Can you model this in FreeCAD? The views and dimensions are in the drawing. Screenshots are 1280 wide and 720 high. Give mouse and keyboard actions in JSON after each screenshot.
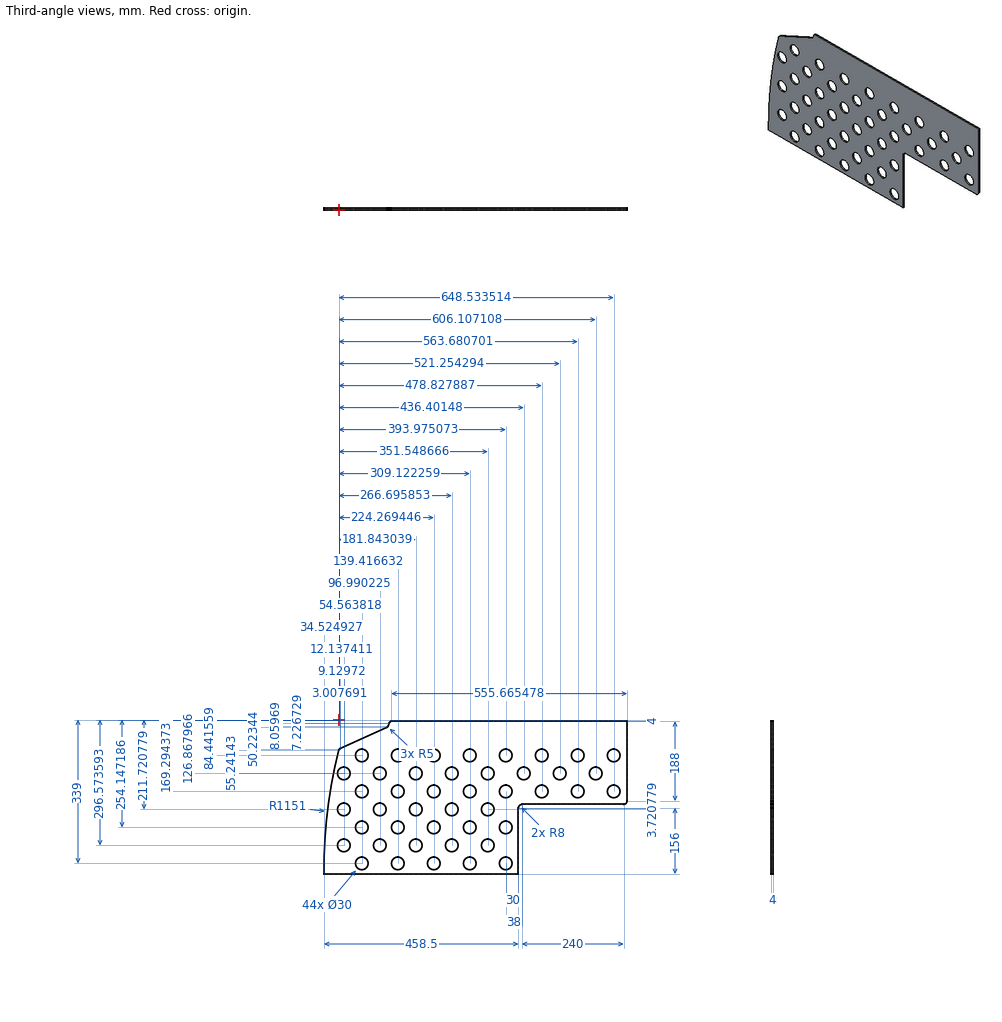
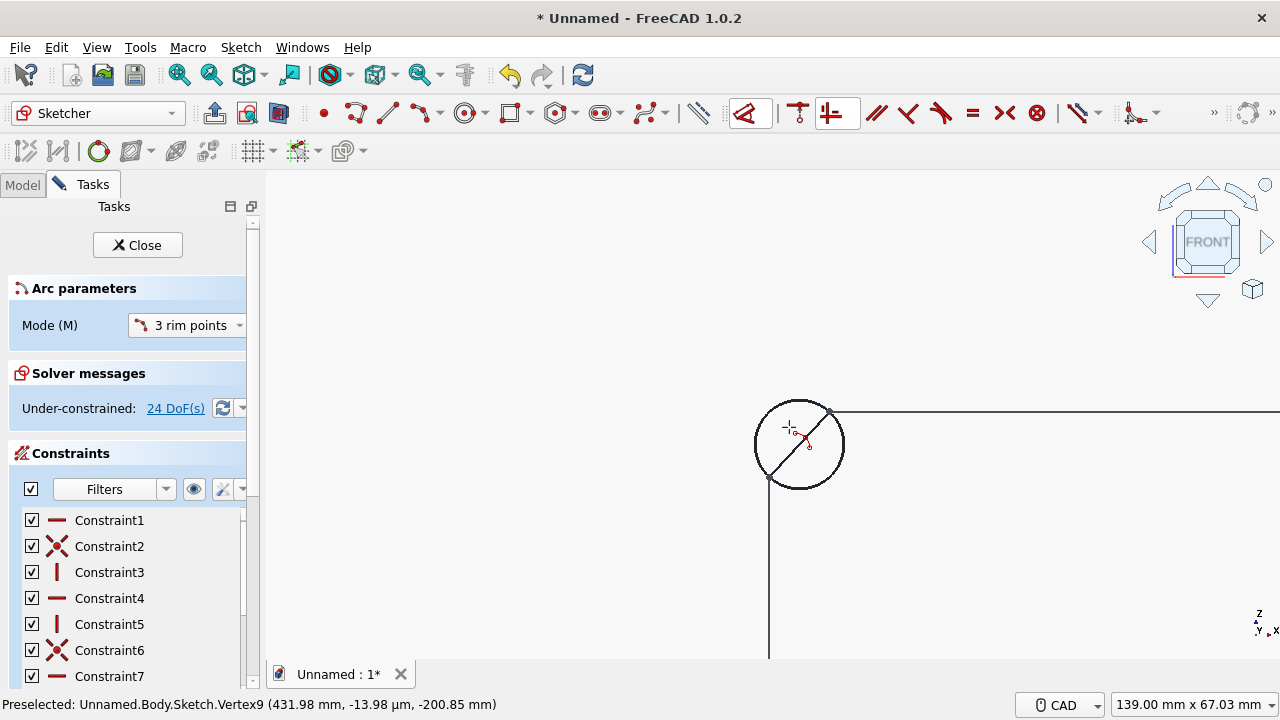
{"action": "left_click", "coordinate": [788, 423]}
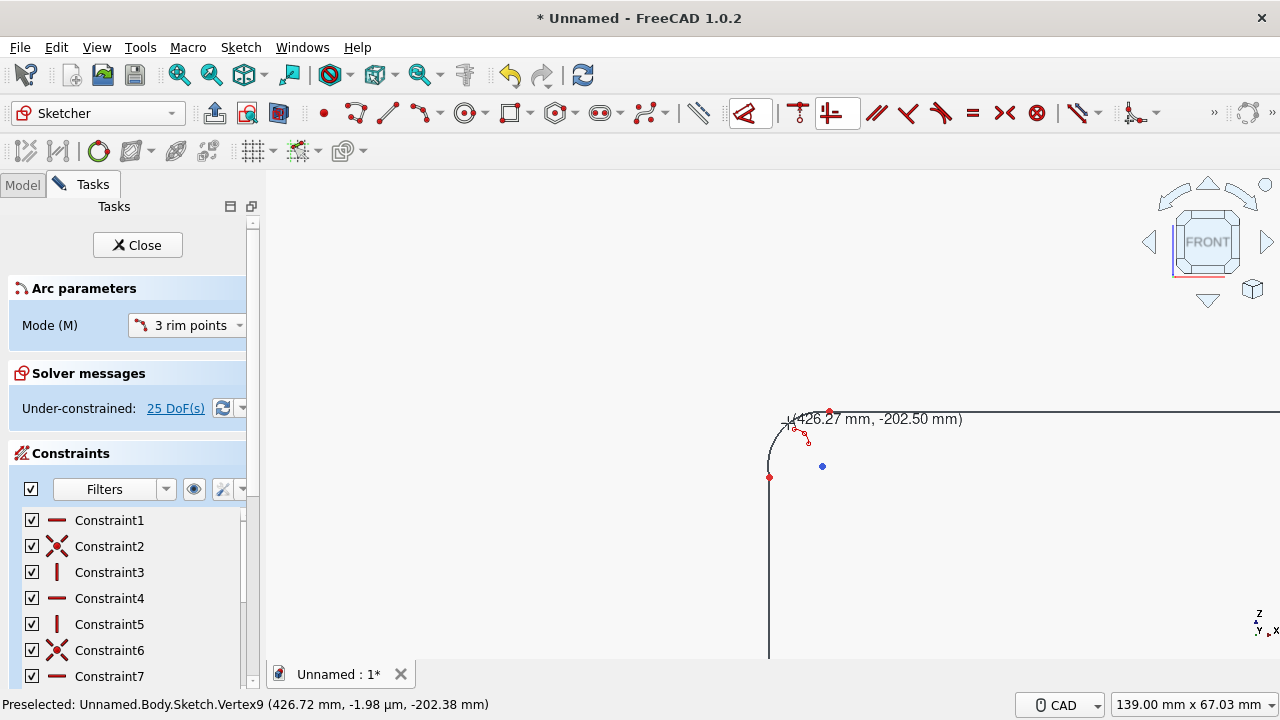
{"action": "scroll", "coordinate": [788, 432], "scroll_direction": "down", "scroll_amount": 11}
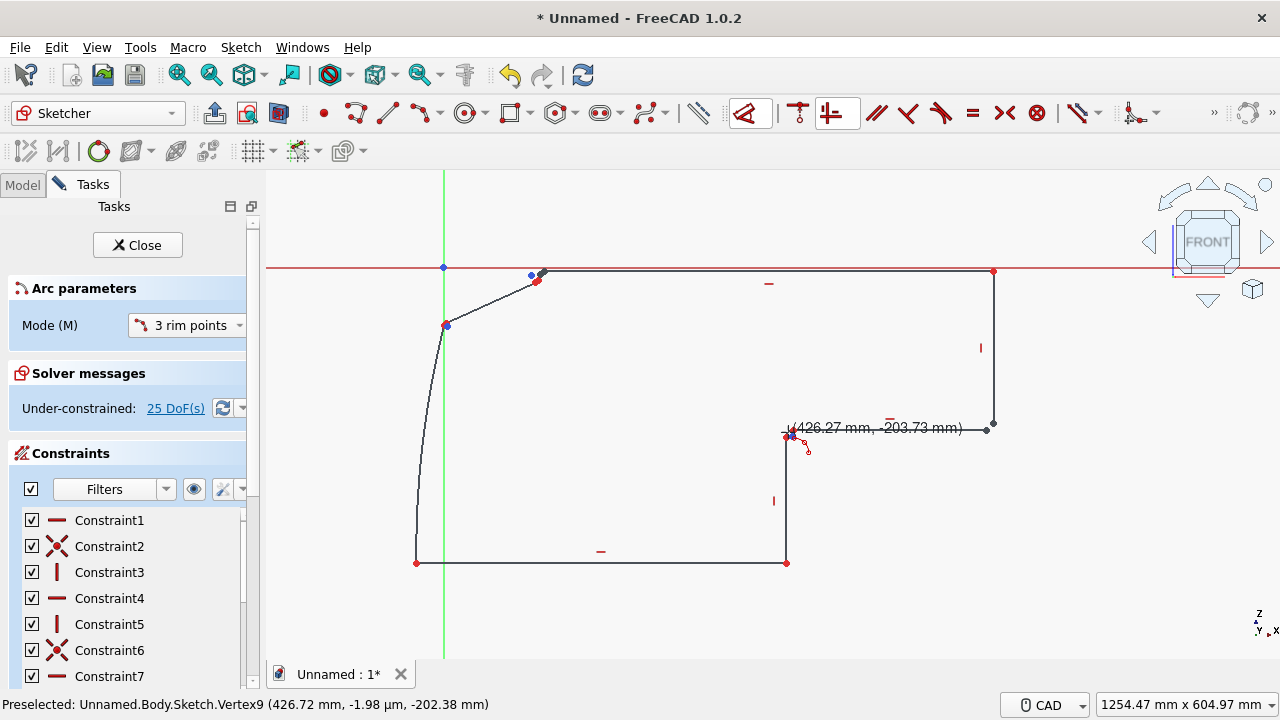
{"action": "scroll", "coordinate": [987, 430], "scroll_direction": "up", "scroll_amount": 3}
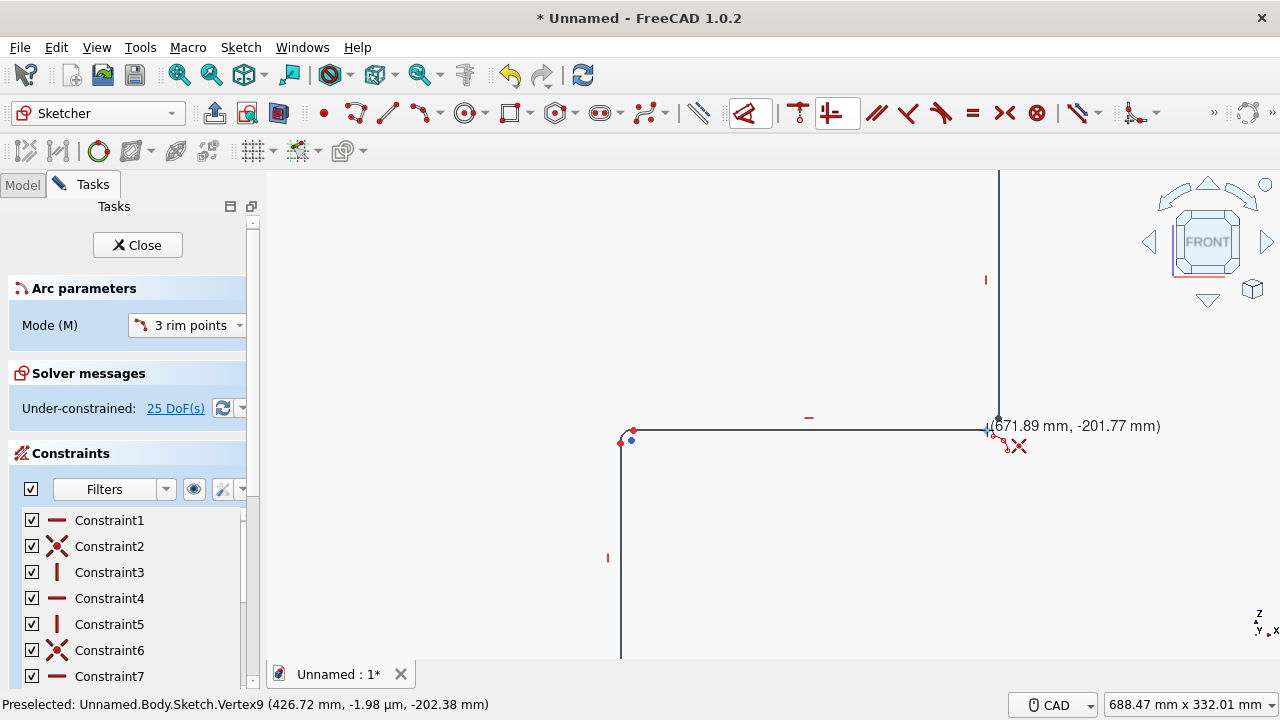
{"action": "left_click", "coordinate": [986, 430]}
{"action": "left_click", "coordinate": [999, 418]}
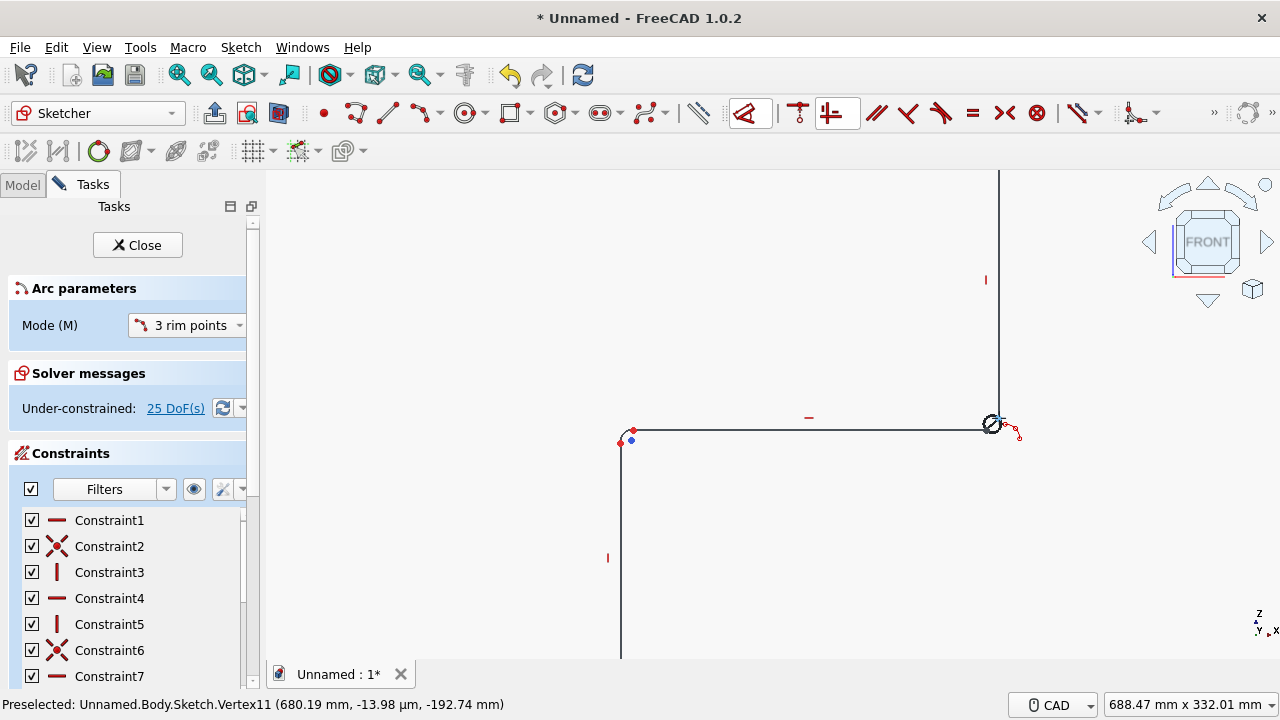
{"action": "scroll", "coordinate": [995, 425], "scroll_direction": "up", "scroll_amount": 8}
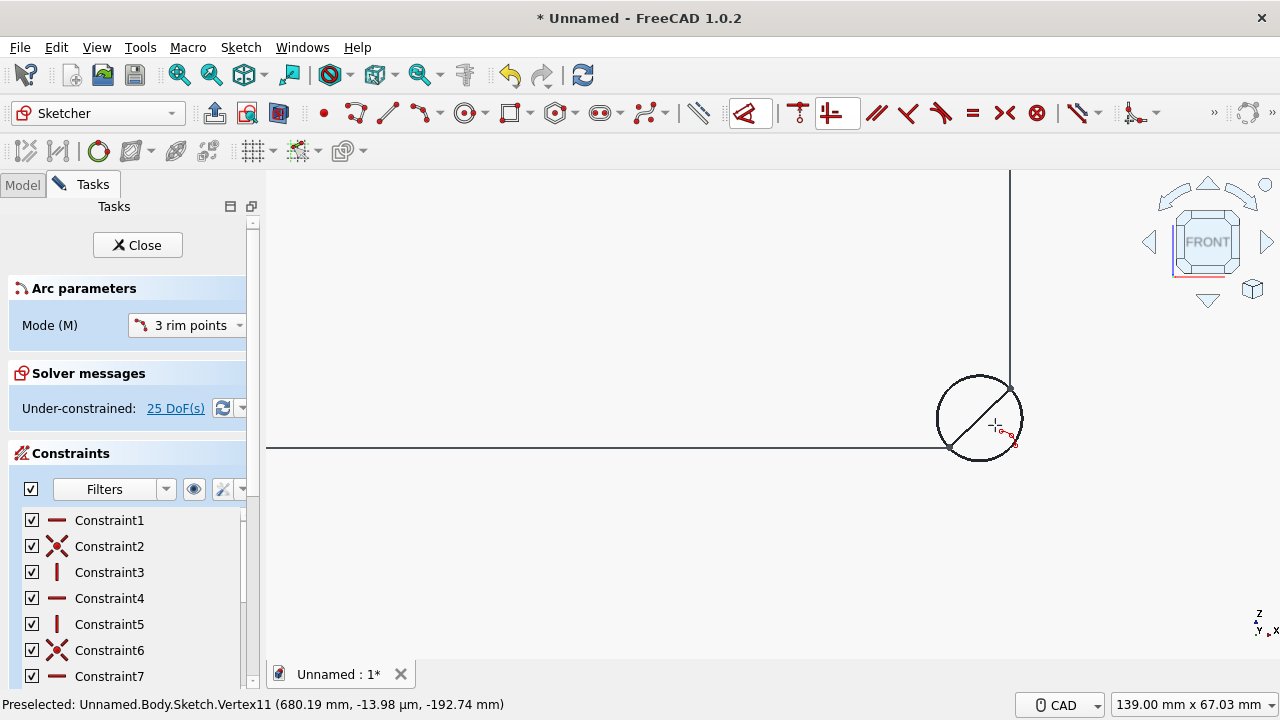
{"action": "left_click", "coordinate": [992, 425]}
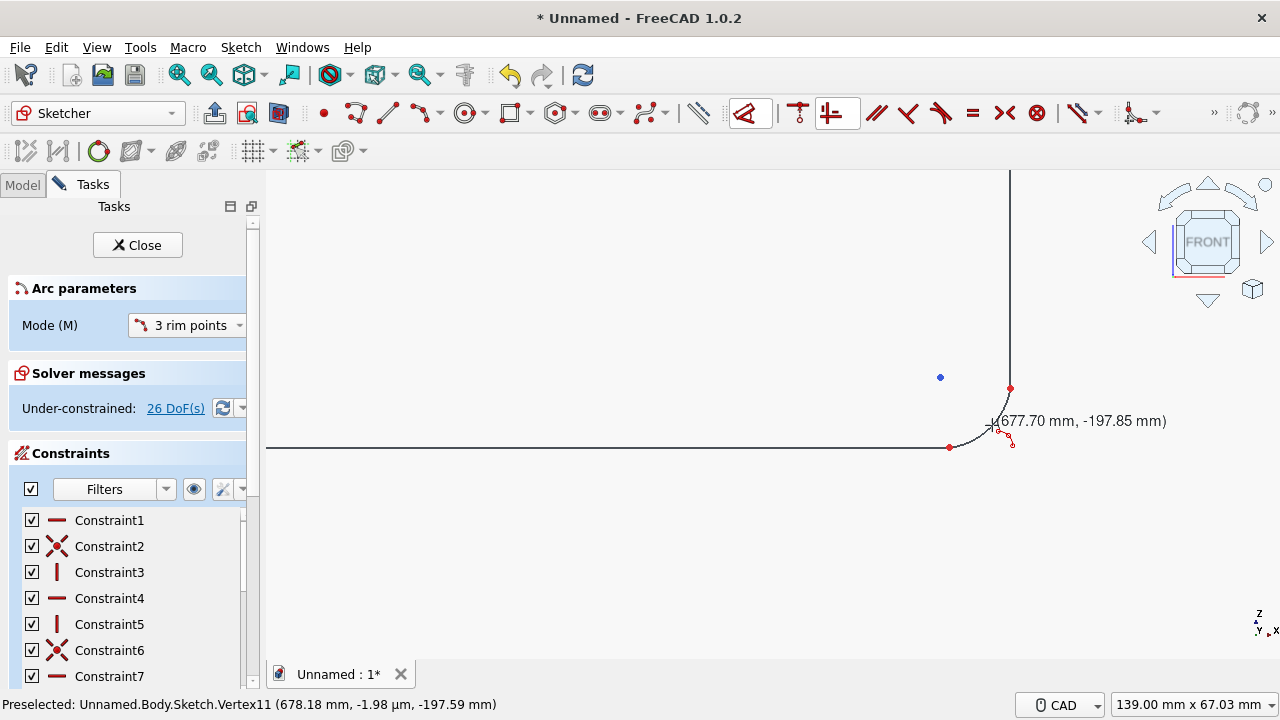
{"action": "scroll", "coordinate": [991, 427], "scroll_direction": "down", "scroll_amount": 11}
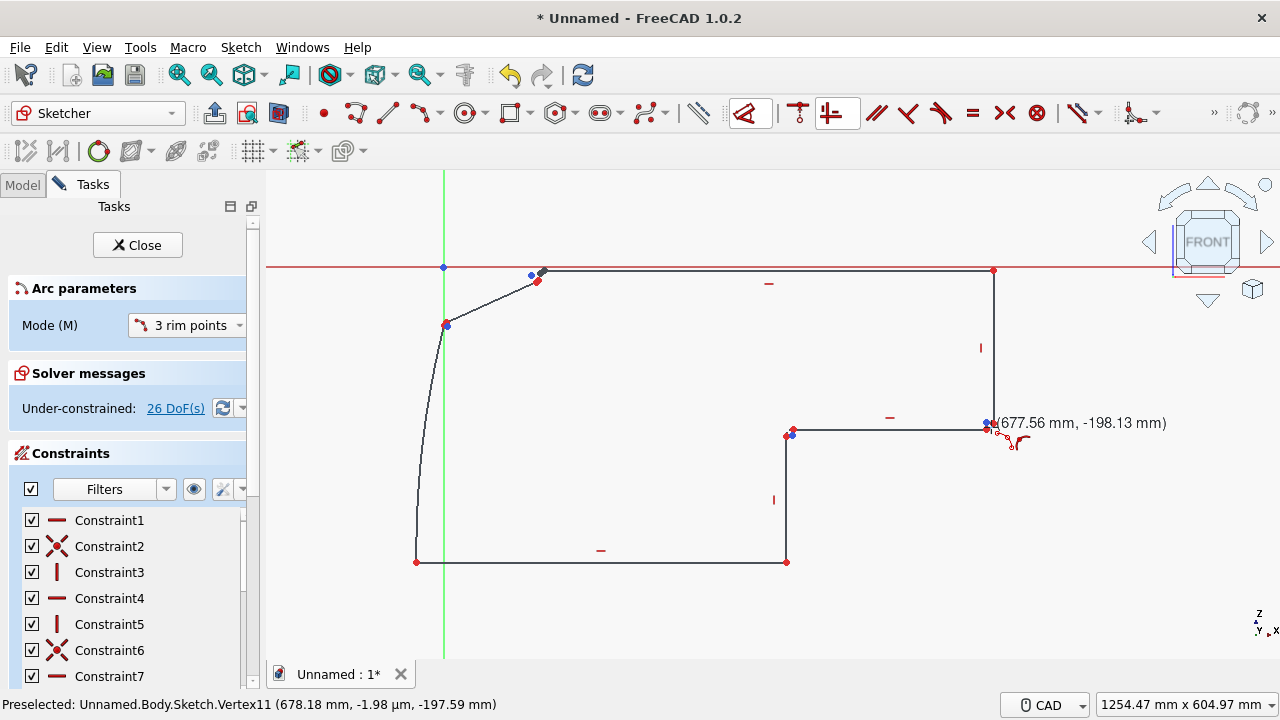
{"action": "scroll", "coordinate": [544, 271], "scroll_direction": "up", "scroll_amount": 8}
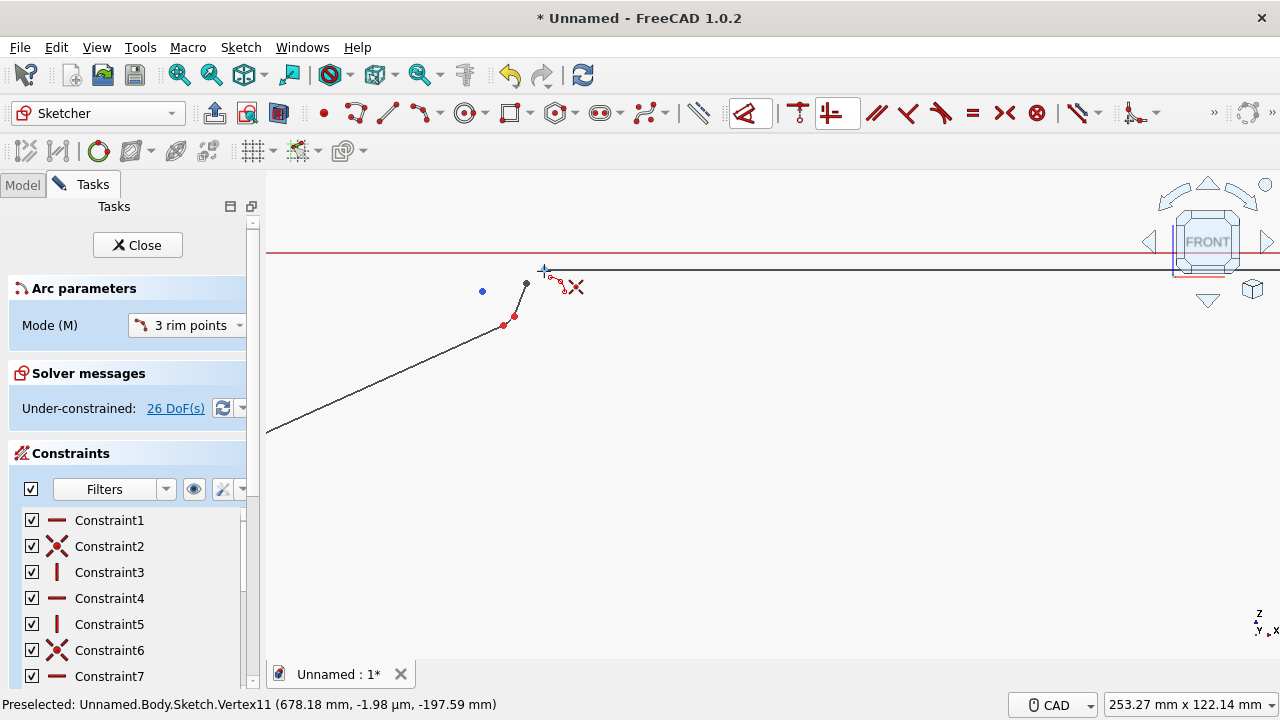
{"action": "left_click", "coordinate": [545, 270]}
{"action": "left_click", "coordinate": [527, 283]}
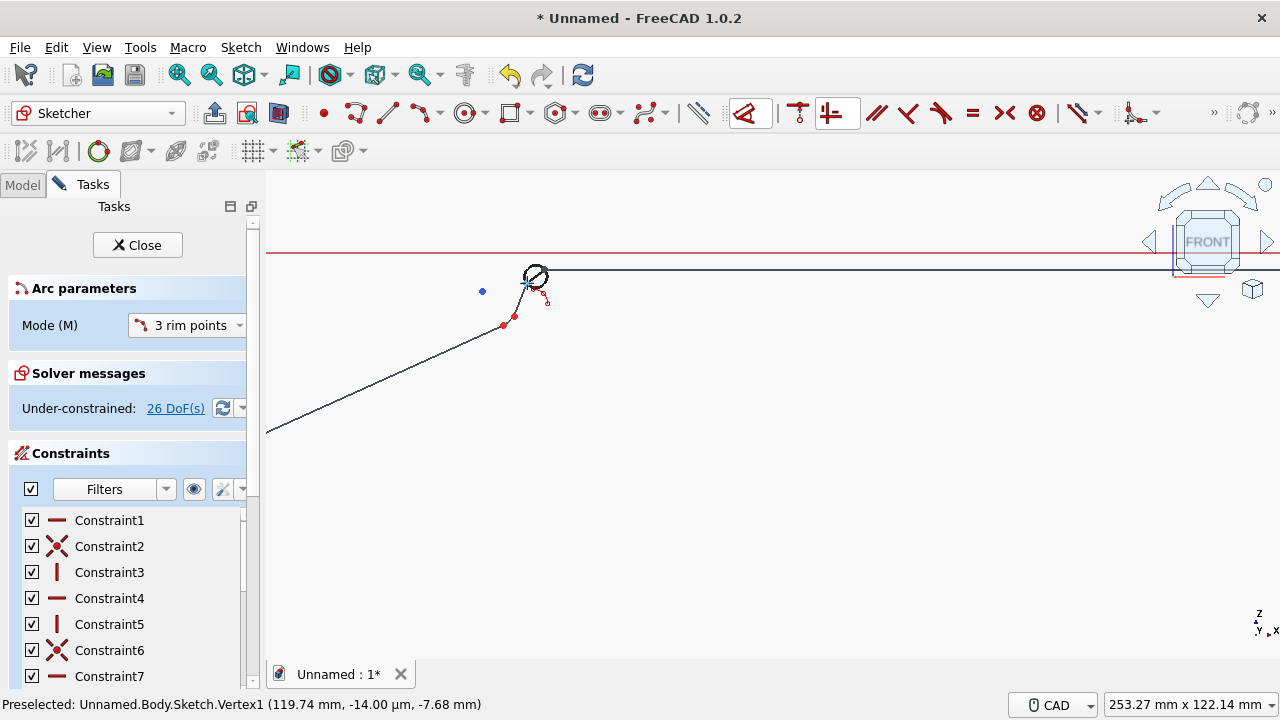
{"action": "scroll", "coordinate": [534, 272], "scroll_direction": "up", "scroll_amount": 8}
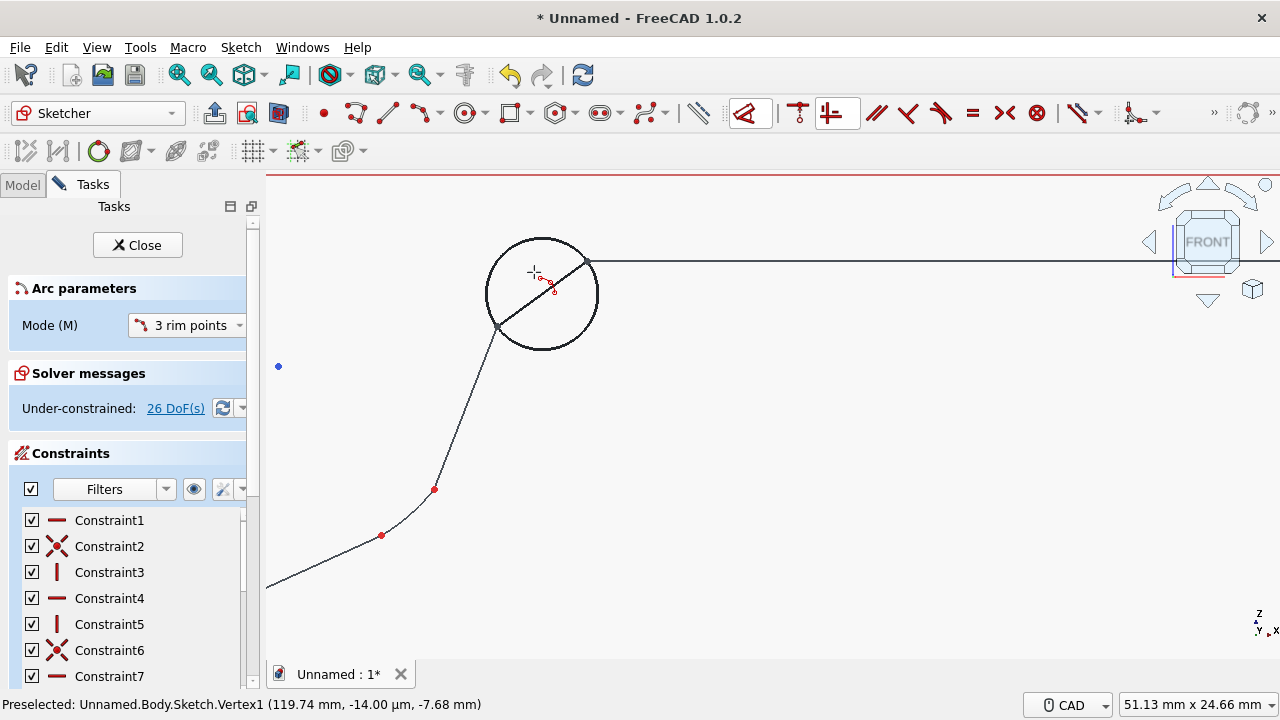
{"action": "left_click", "coordinate": [532, 271]}